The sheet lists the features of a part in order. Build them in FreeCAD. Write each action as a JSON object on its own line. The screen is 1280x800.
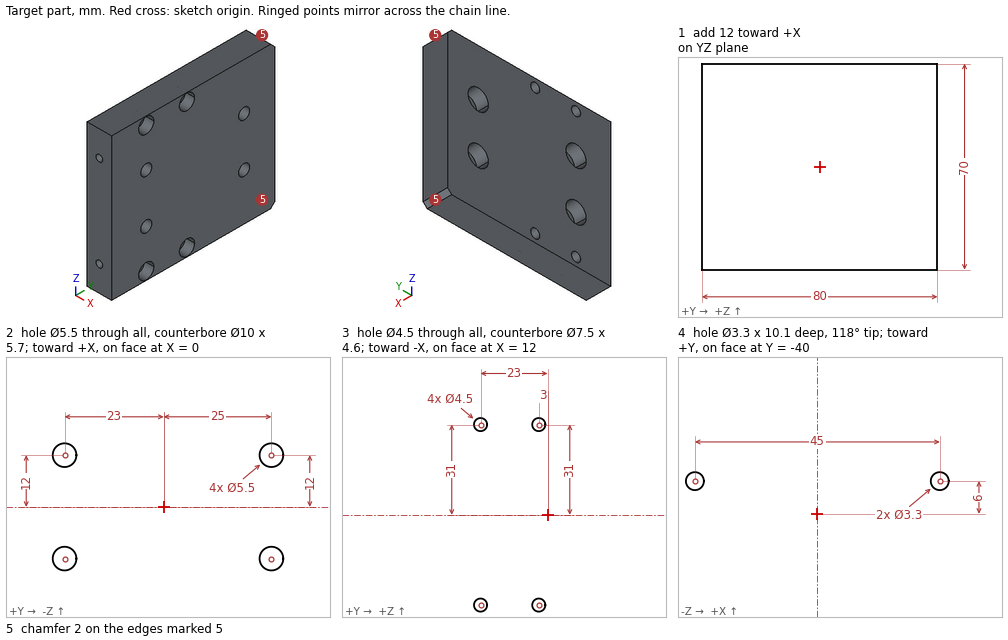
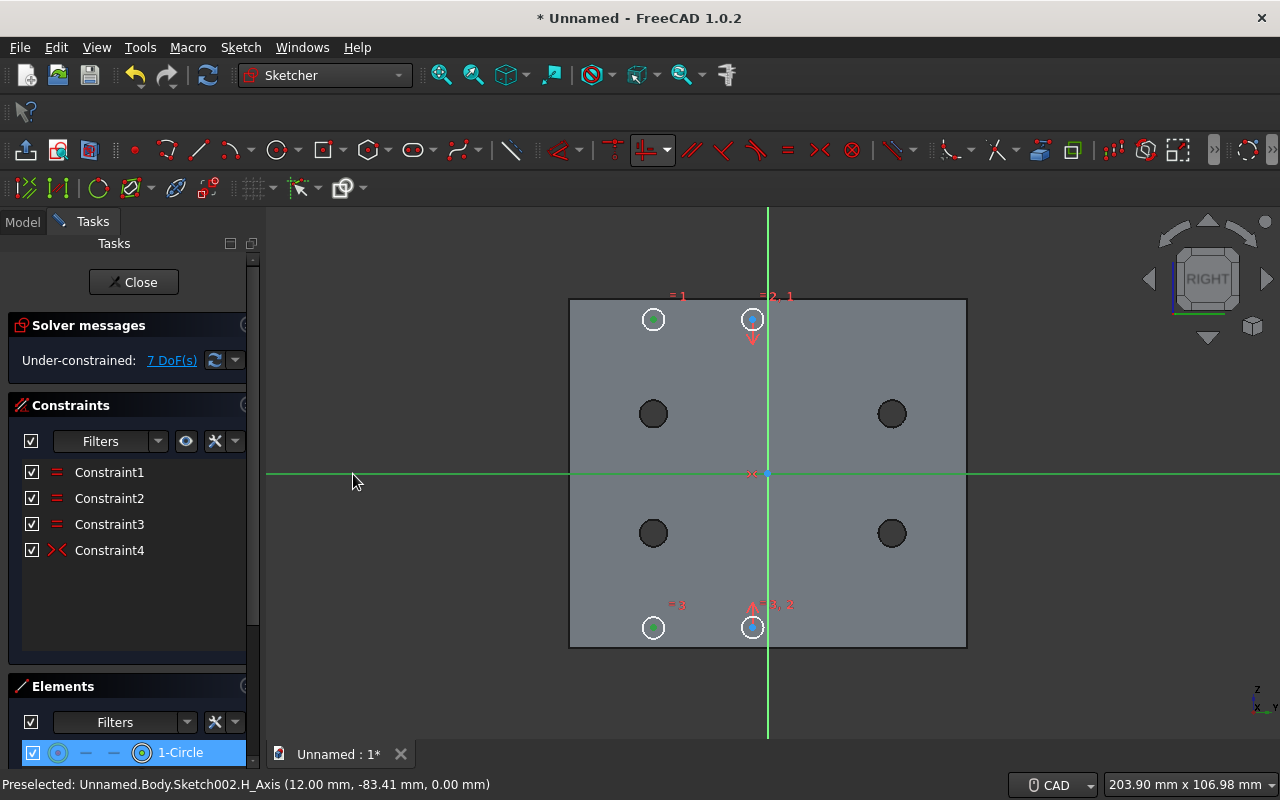
{"action": "left_click", "coordinate": [820, 150]}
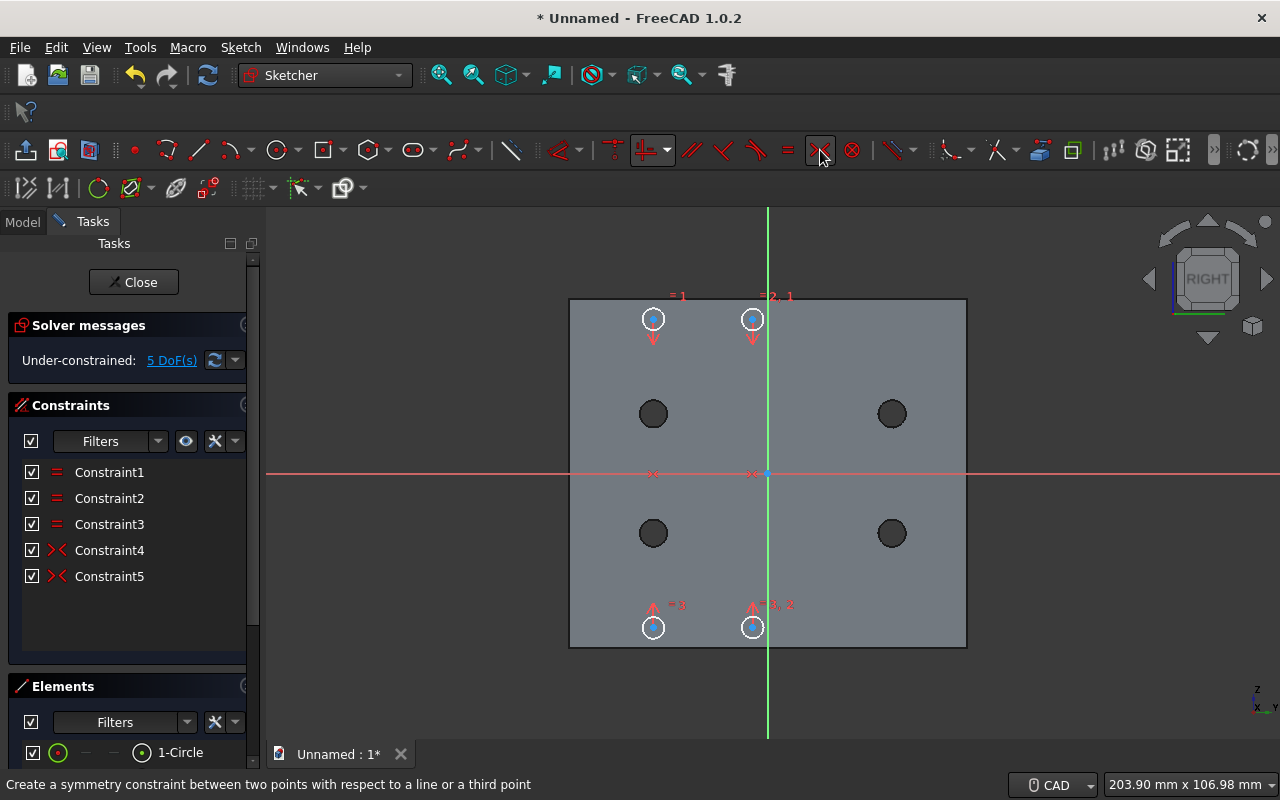
{"action": "left_click", "coordinate": [558, 150]}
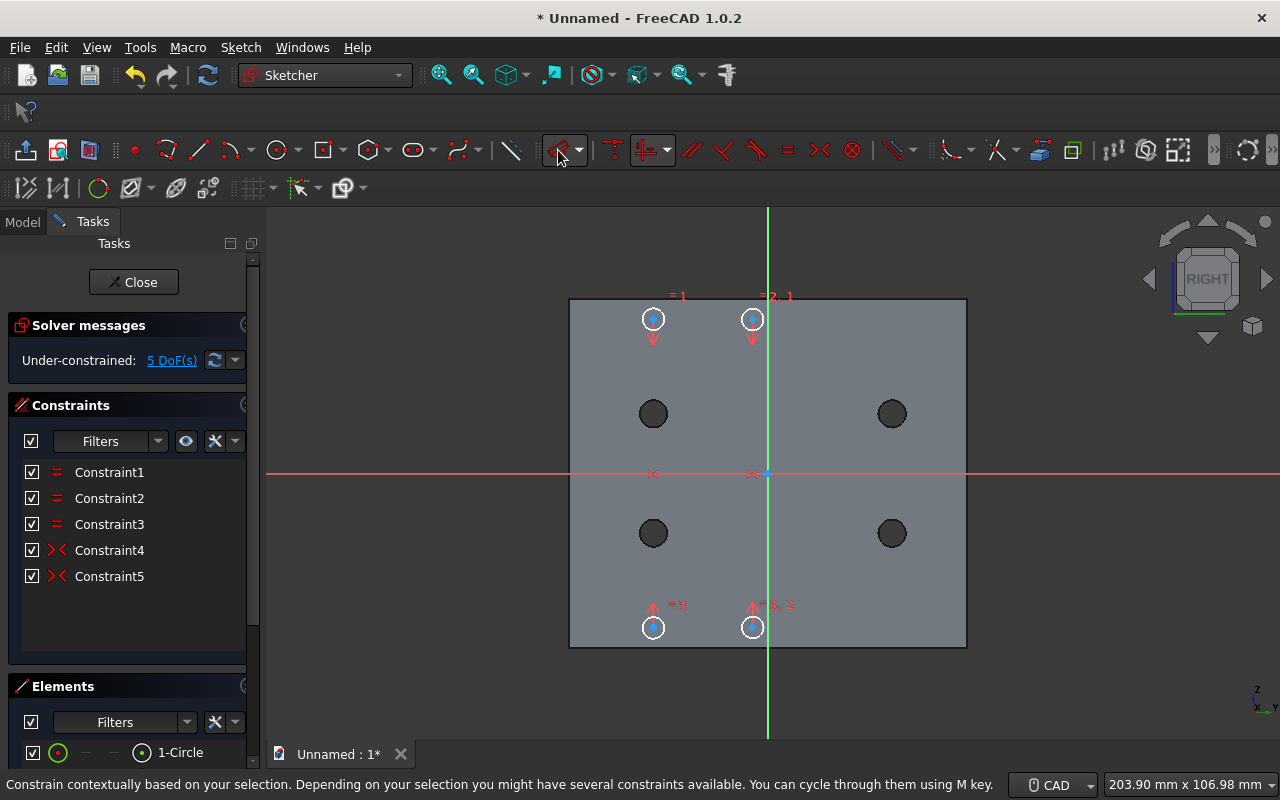
{"action": "scroll", "coordinate": [661, 312], "scroll_direction": "up", "scroll_amount": 3}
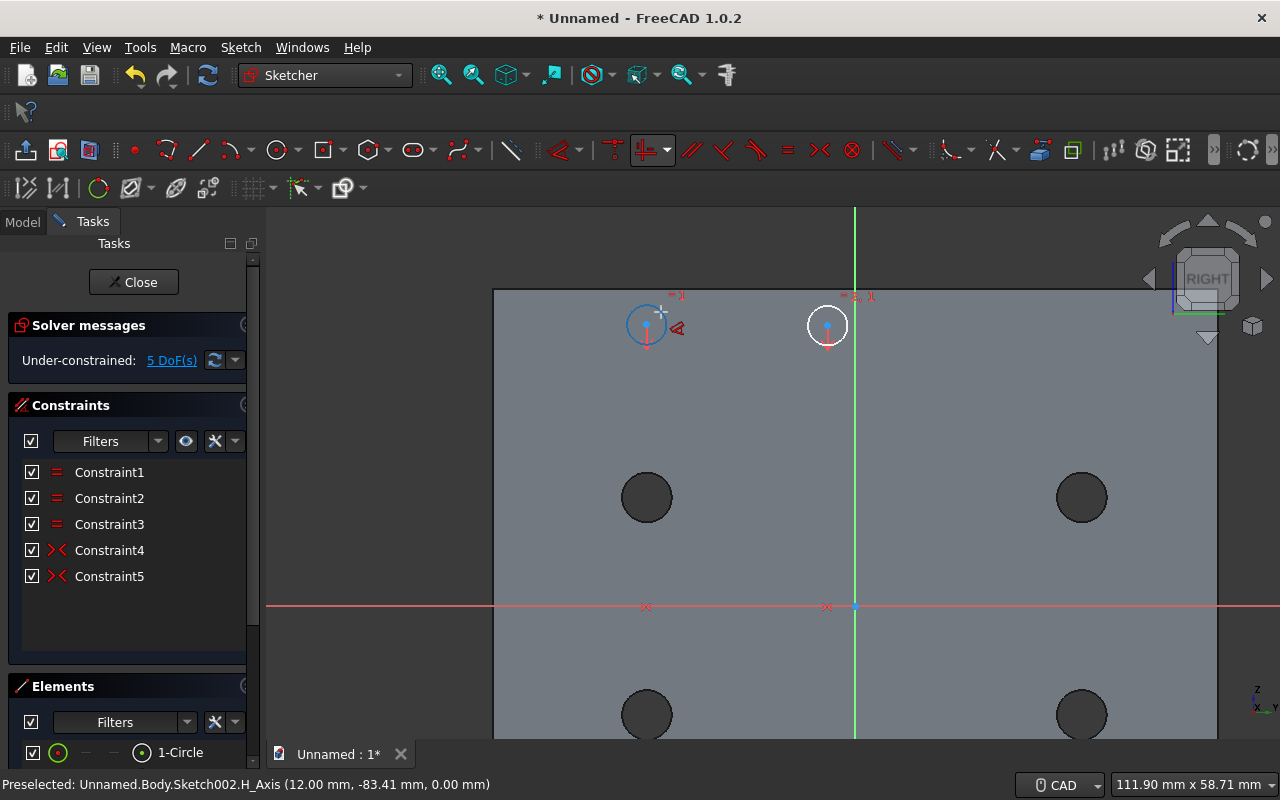
{"action": "left_click", "coordinate": [661, 311]}
{"action": "left_click", "coordinate": [684, 289]}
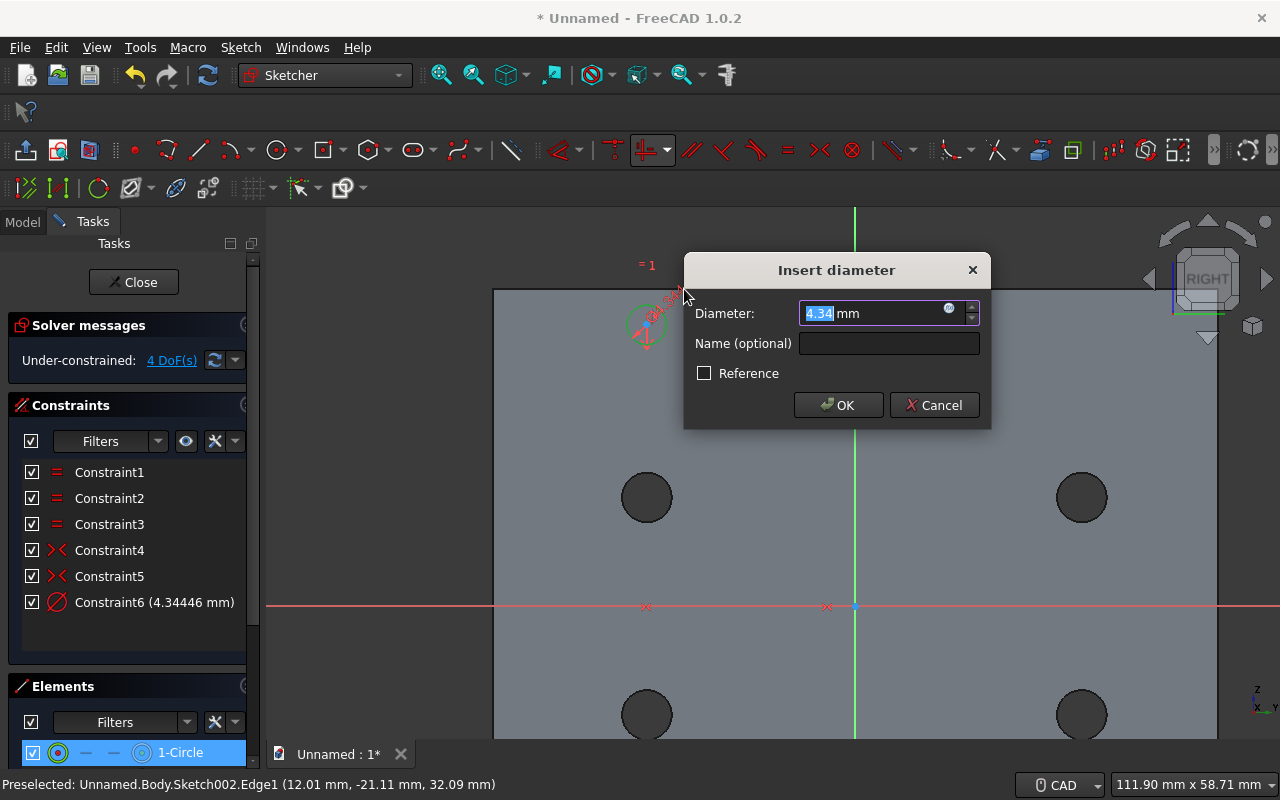
{"action": "type", "text": "4.5"}
{"action": "key", "text": "Return"}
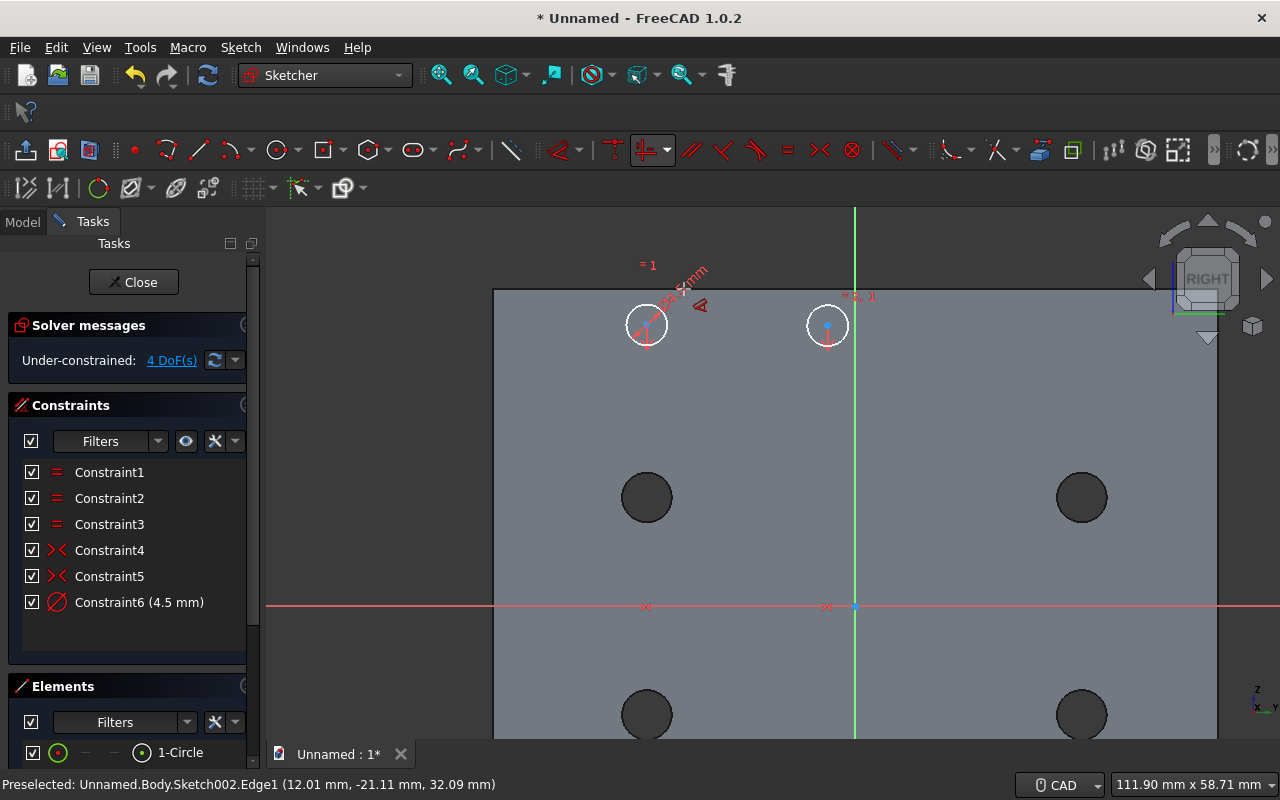
{"action": "scroll", "coordinate": [828, 326], "scroll_direction": "up", "scroll_amount": 2}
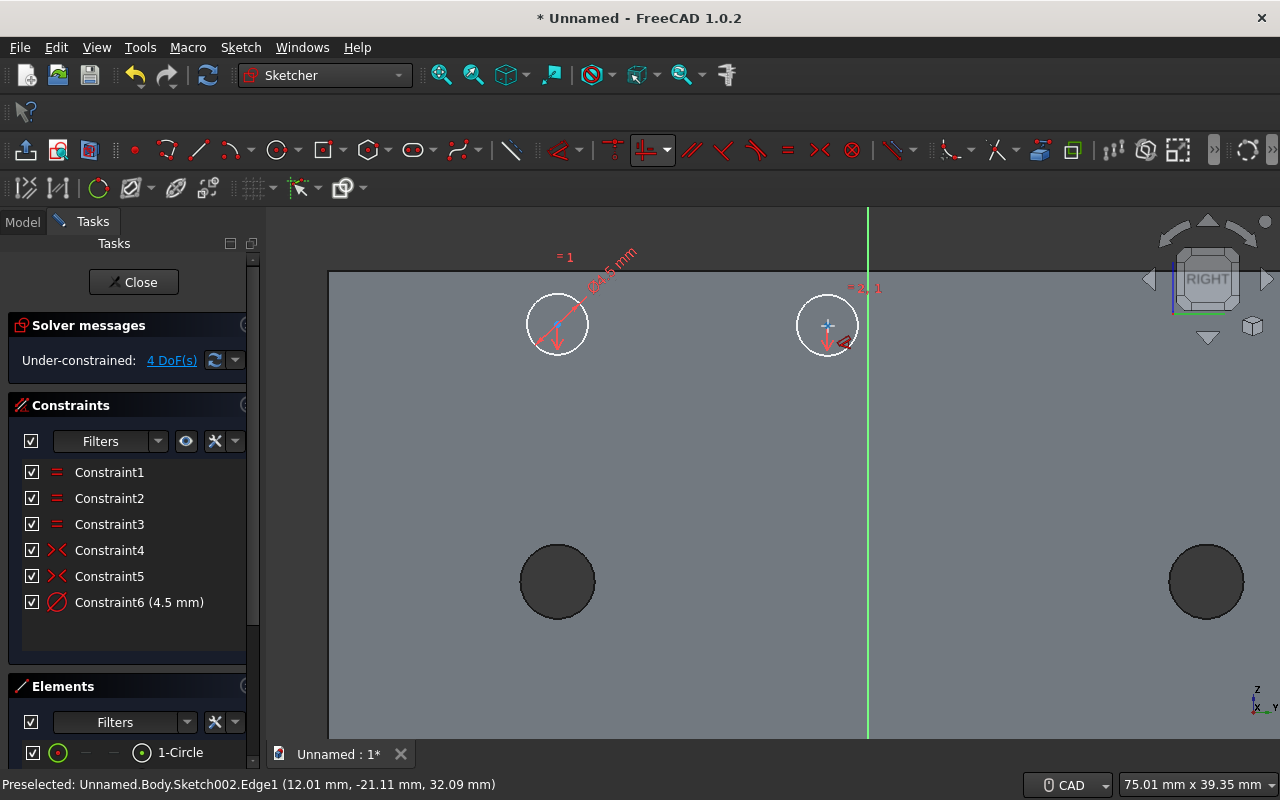
{"action": "left_click", "coordinate": [827, 325]}
{"action": "left_click", "coordinate": [848, 267]}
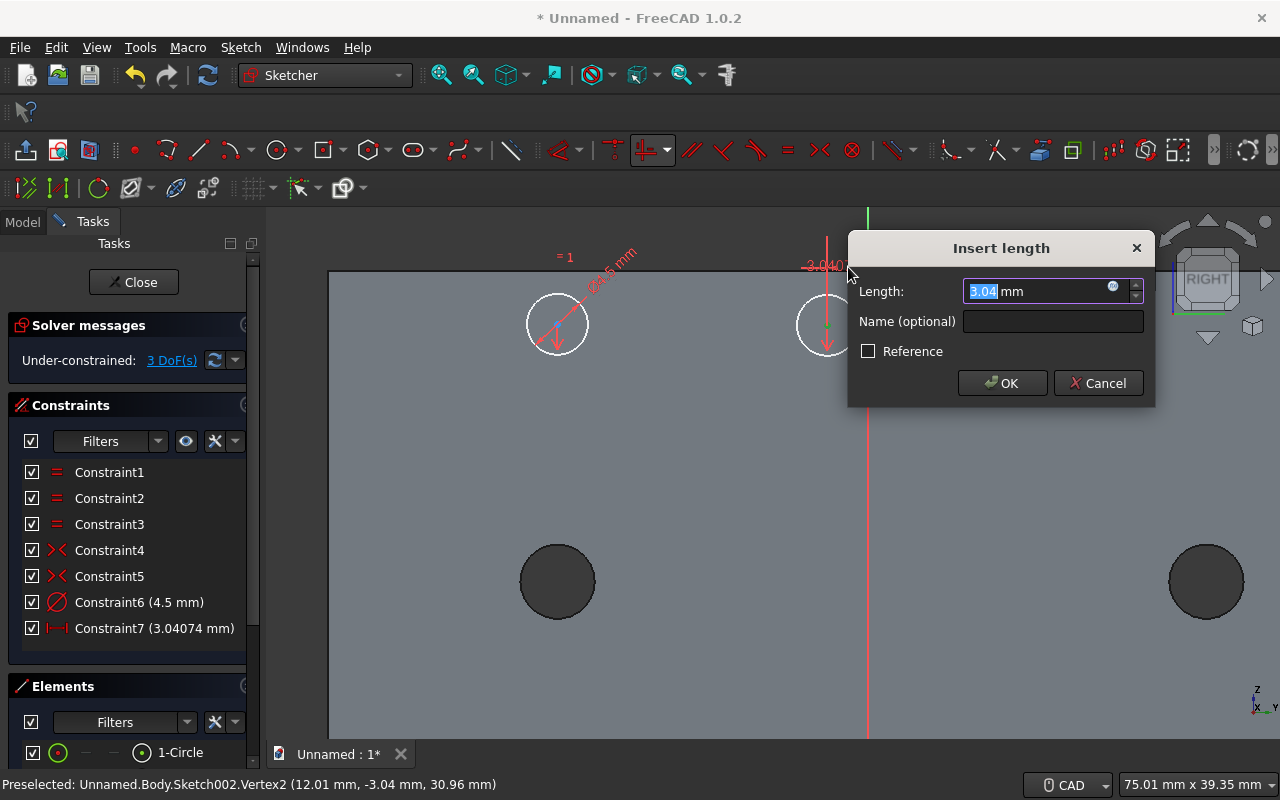
{"action": "type", "text": "3"}
{"action": "key", "text": "Return"}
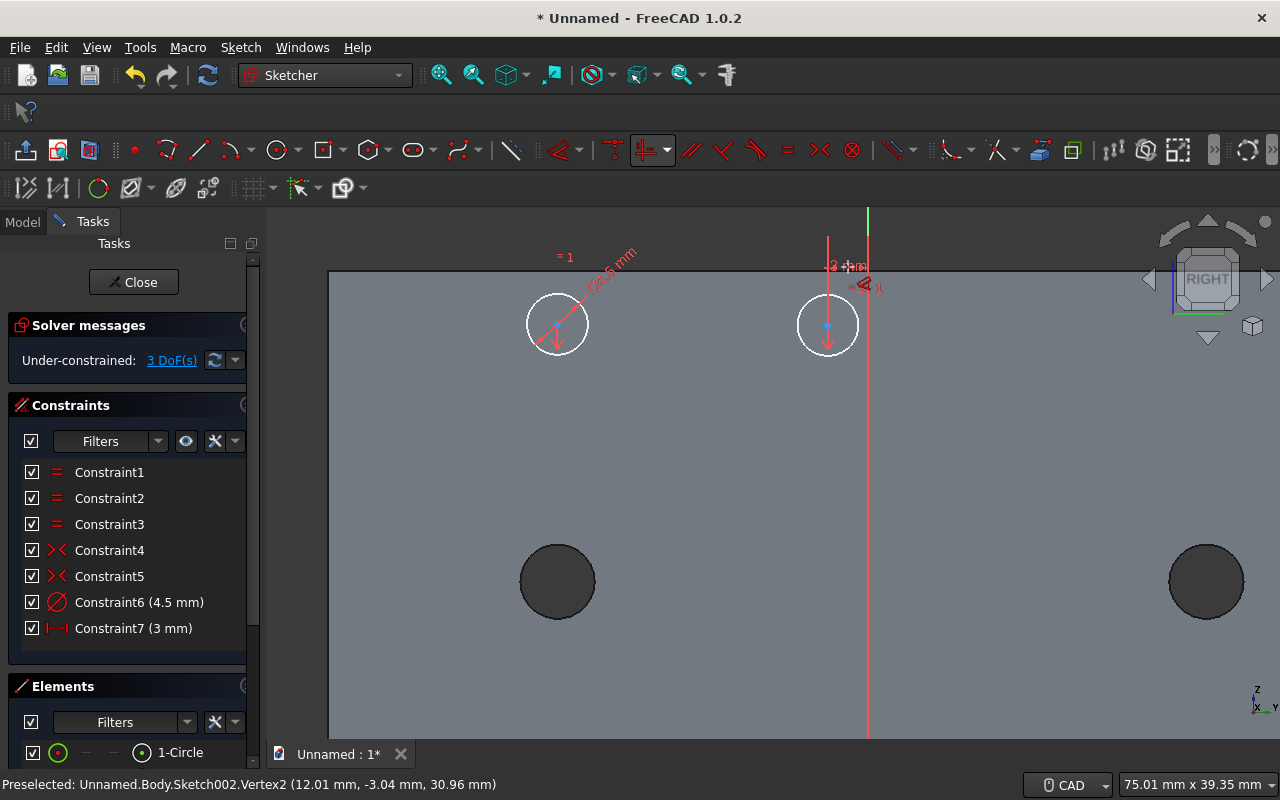
{"action": "left_click", "coordinate": [557, 324]}
{"action": "left_click", "coordinate": [713, 290]}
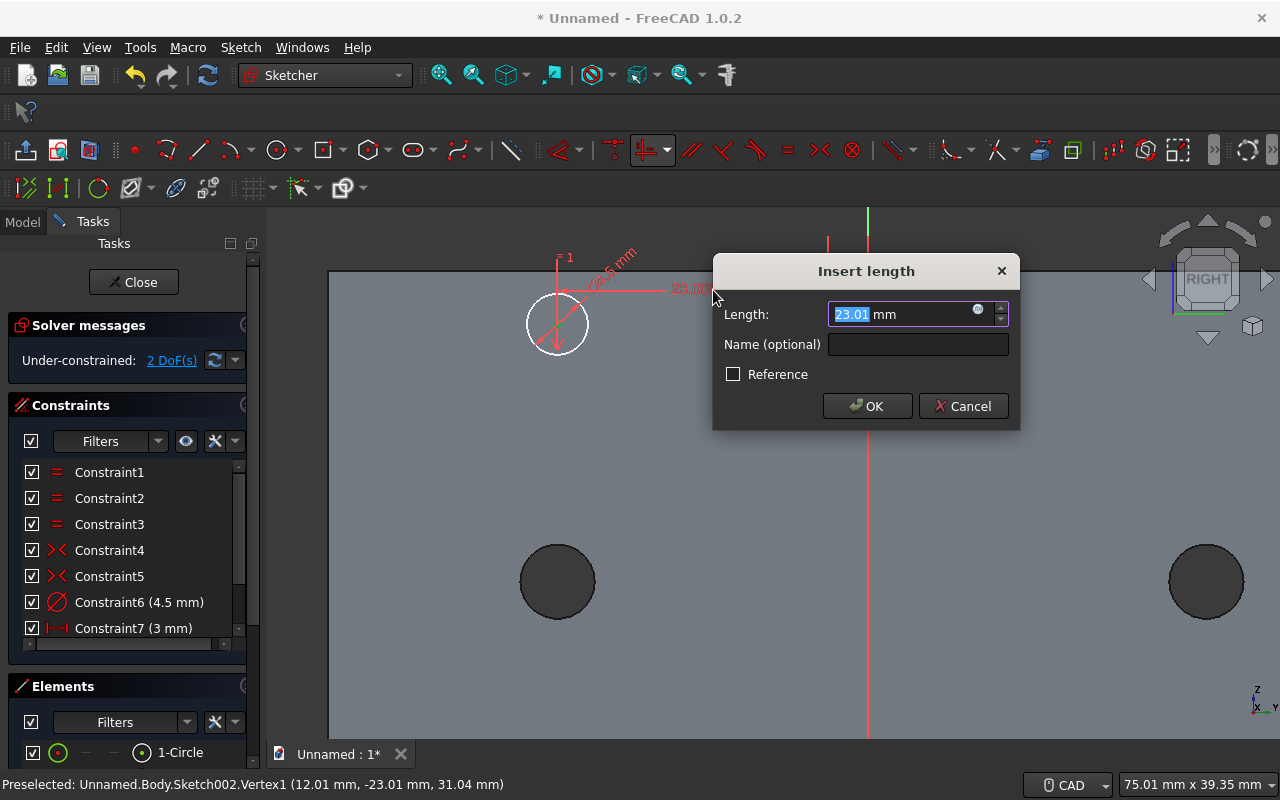
{"action": "type", "text": "23"}
{"action": "key", "text": "Return"}